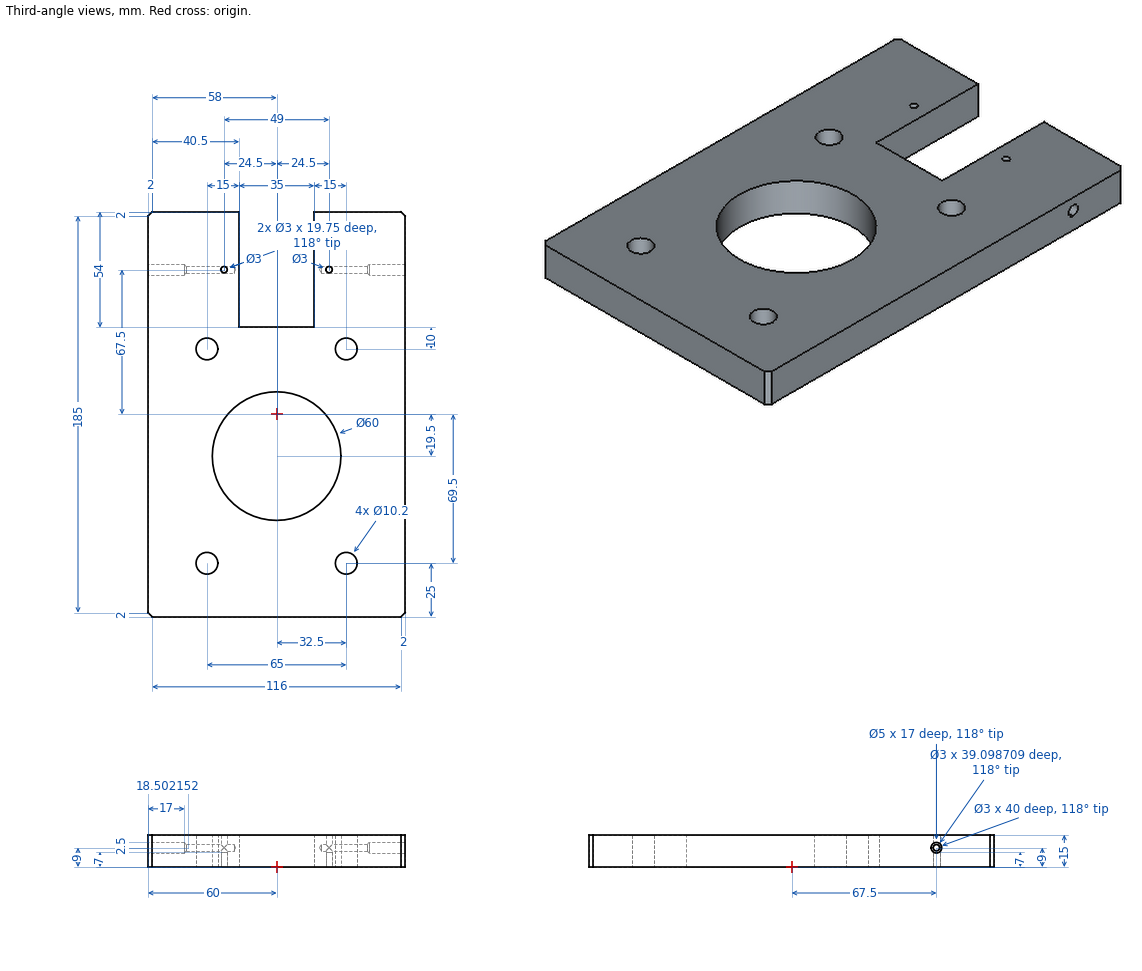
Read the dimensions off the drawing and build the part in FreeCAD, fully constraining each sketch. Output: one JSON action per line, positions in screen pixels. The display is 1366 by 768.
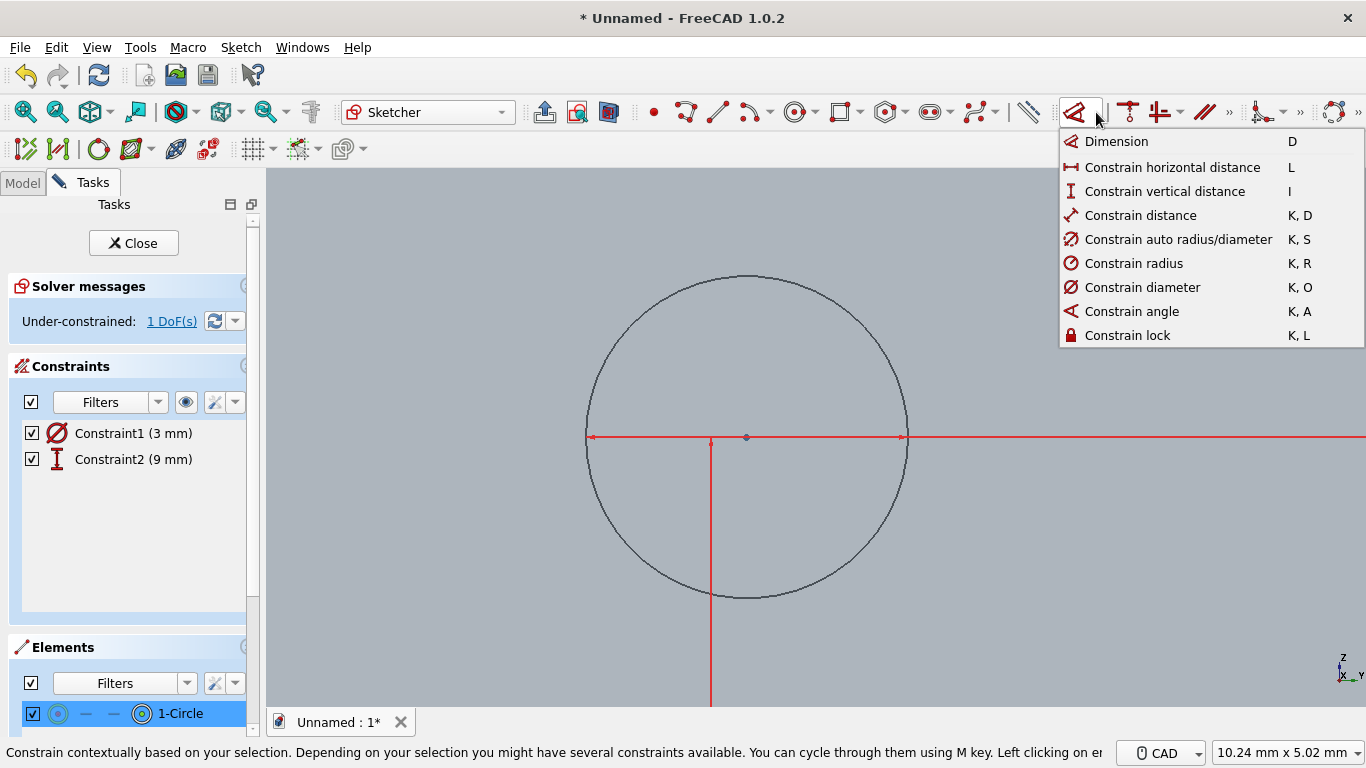
{"action": "left_click", "coordinate": [1212, 167]}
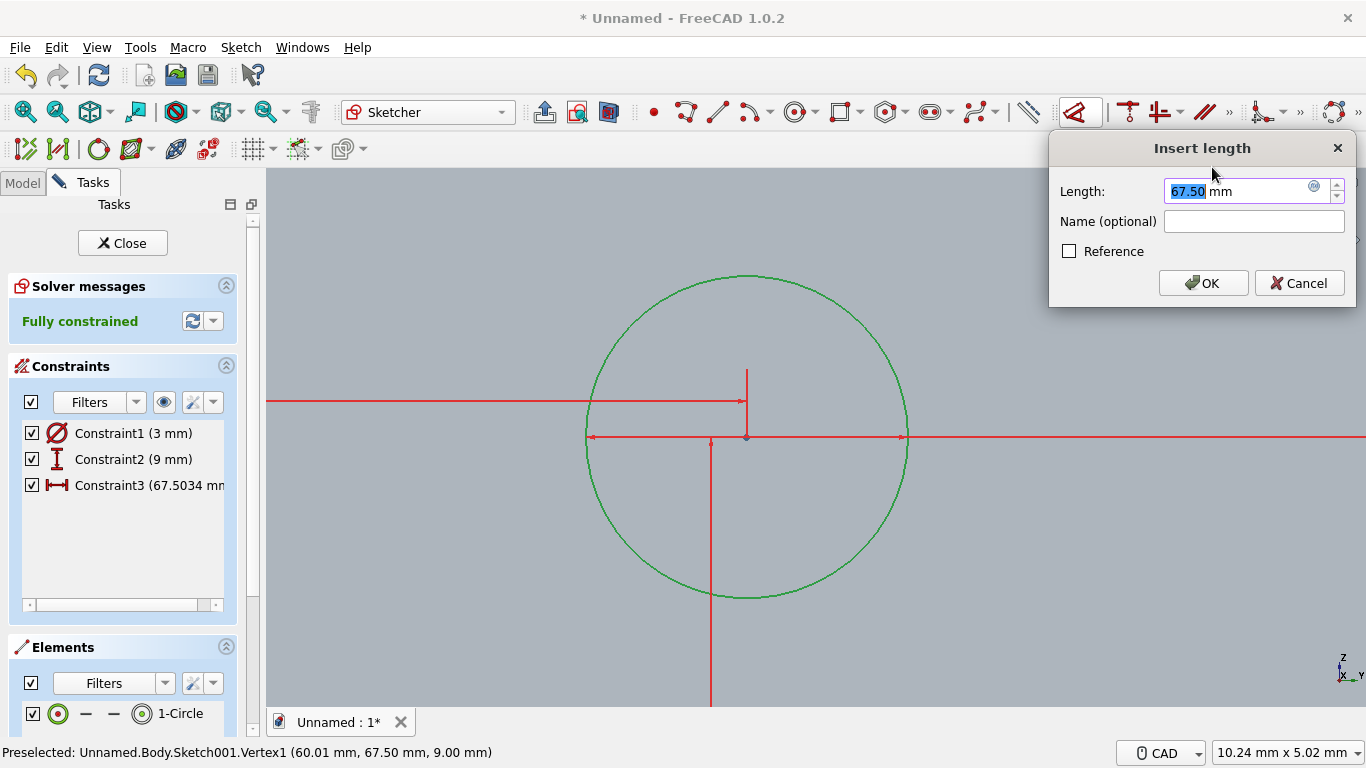
{"action": "type", "text": "67.5"}
{"action": "key", "text": "Return"}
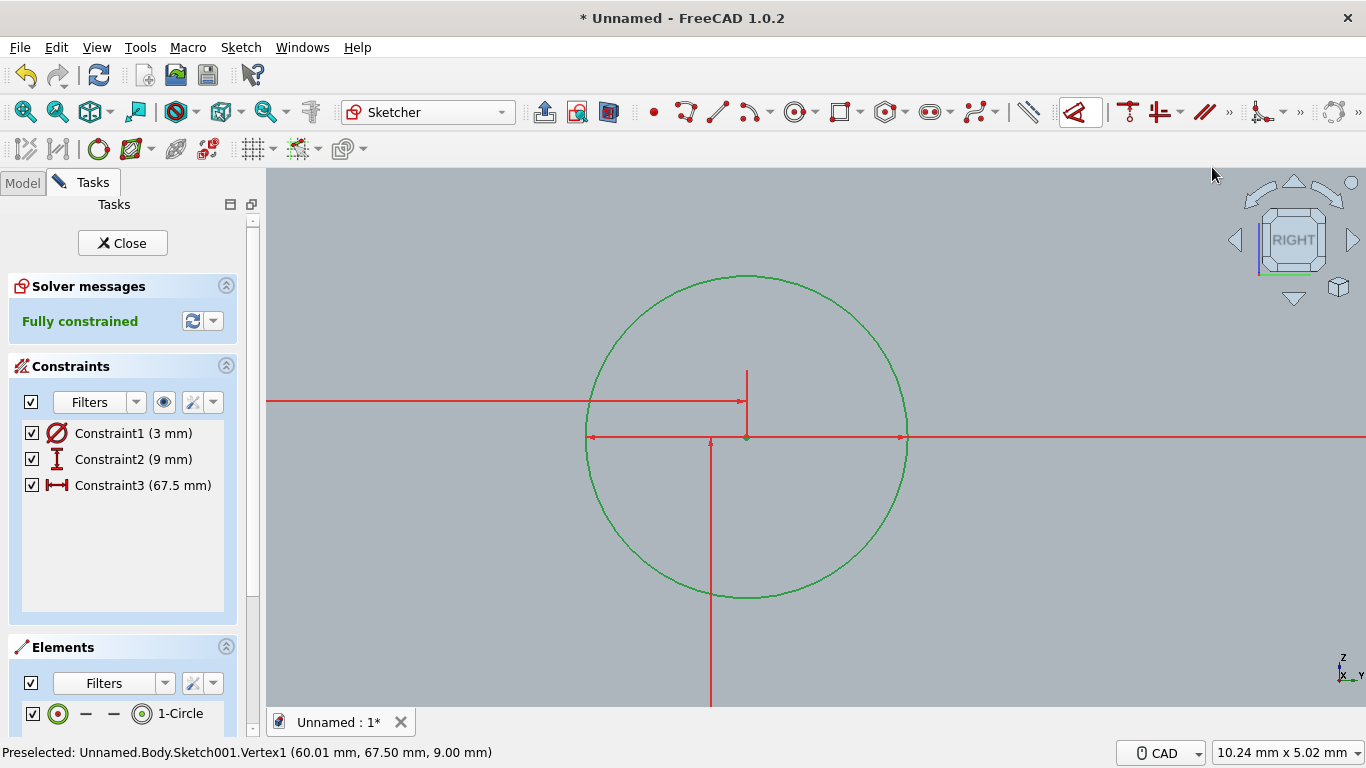
{"action": "left_click", "coordinate": [123, 243]}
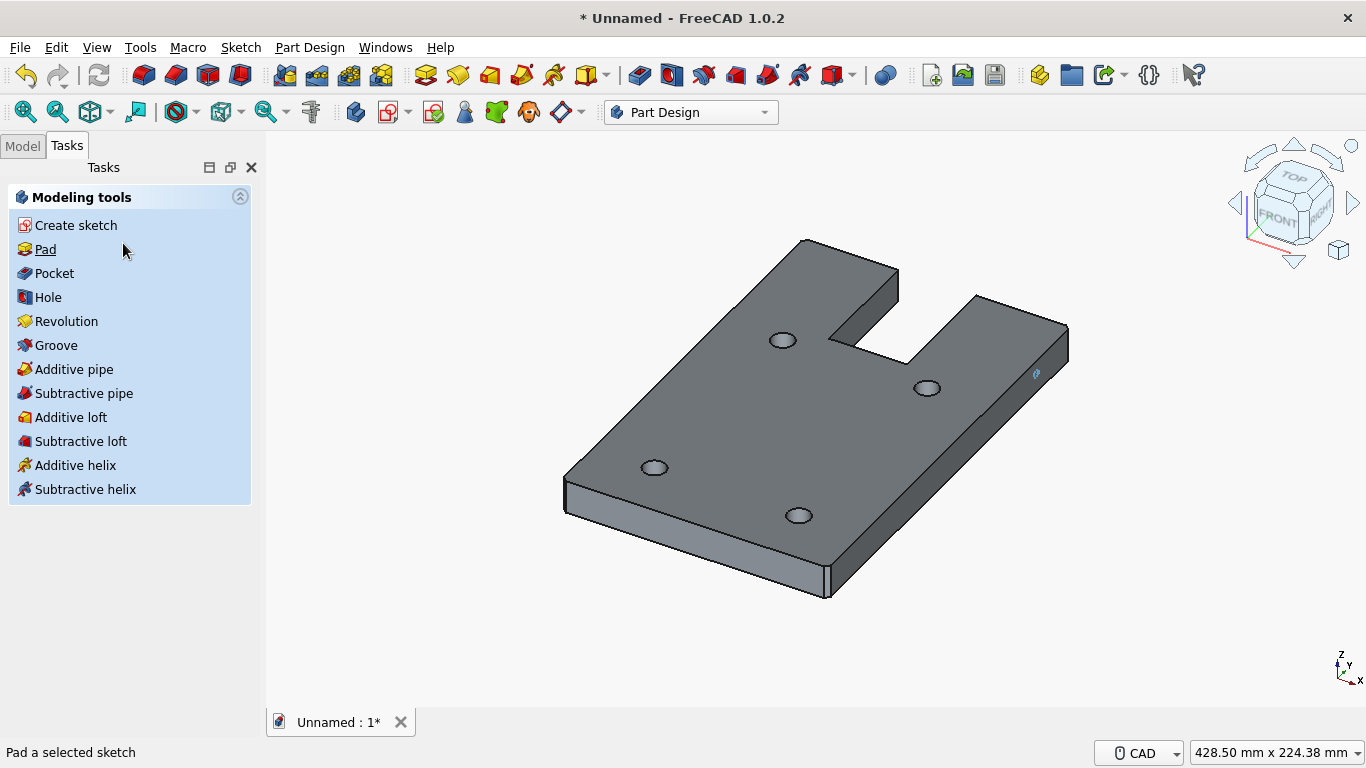
{"action": "left_click", "coordinate": [672, 76]}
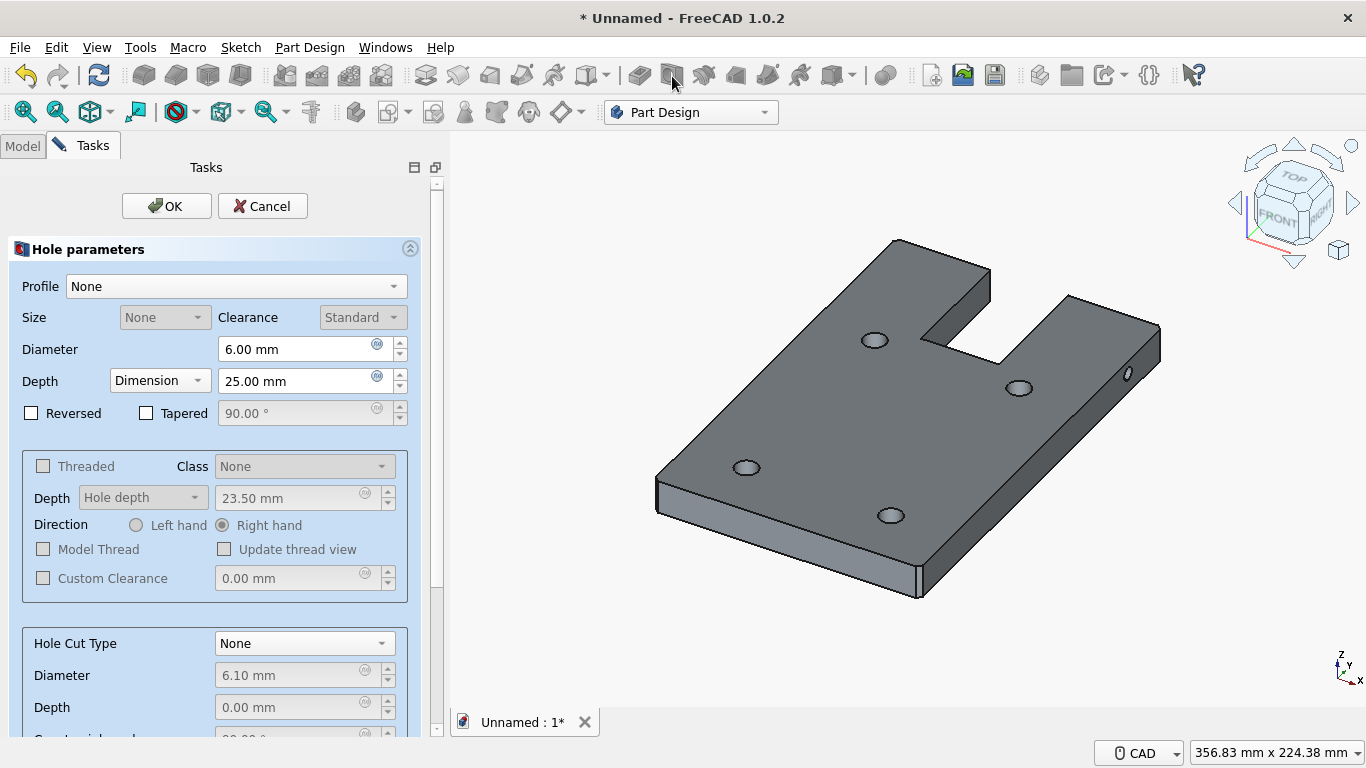
{"action": "triple_click", "coordinate": [305, 349]}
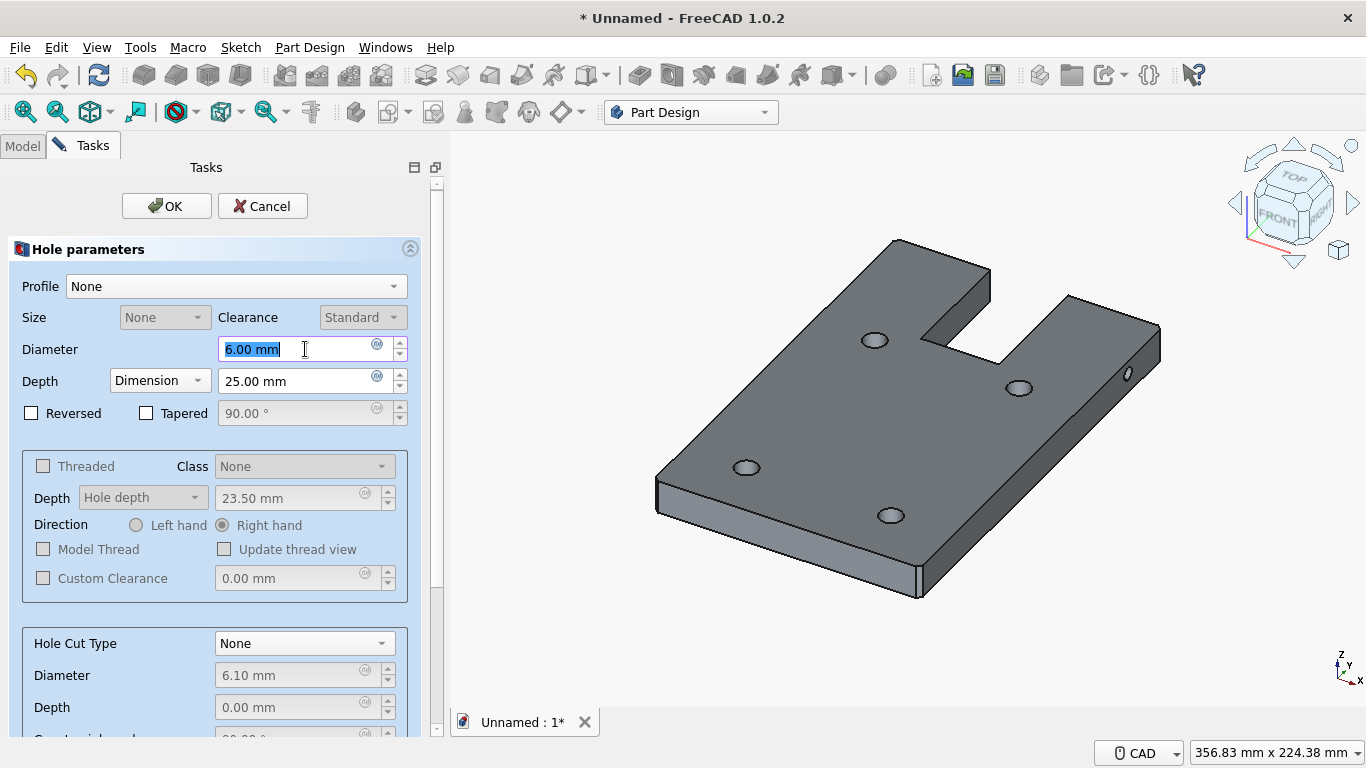
{"action": "type", "text": "3"}
{"action": "key", "text": "Tab"}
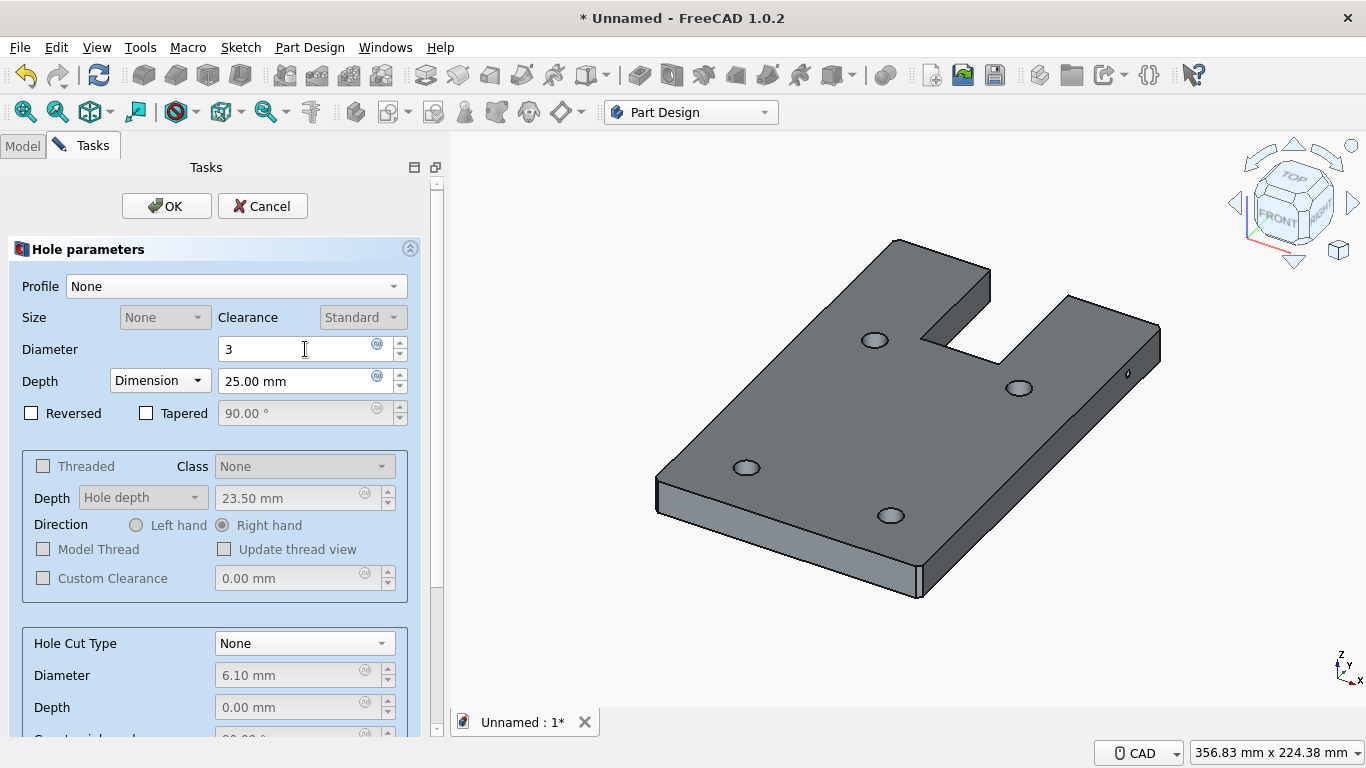
{"action": "triple_click", "coordinate": [305, 381]}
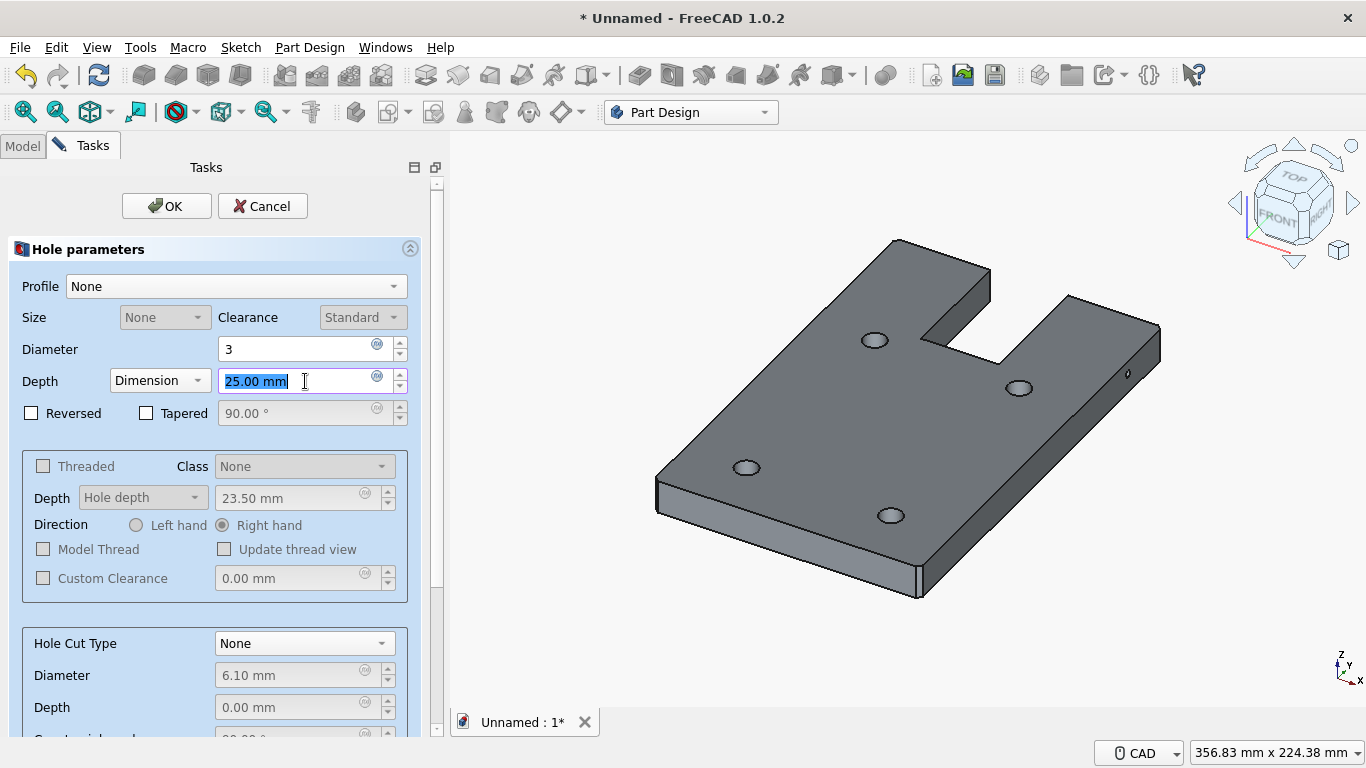
{"action": "type", "text": "39.098709"}
{"action": "key", "text": "Tab"}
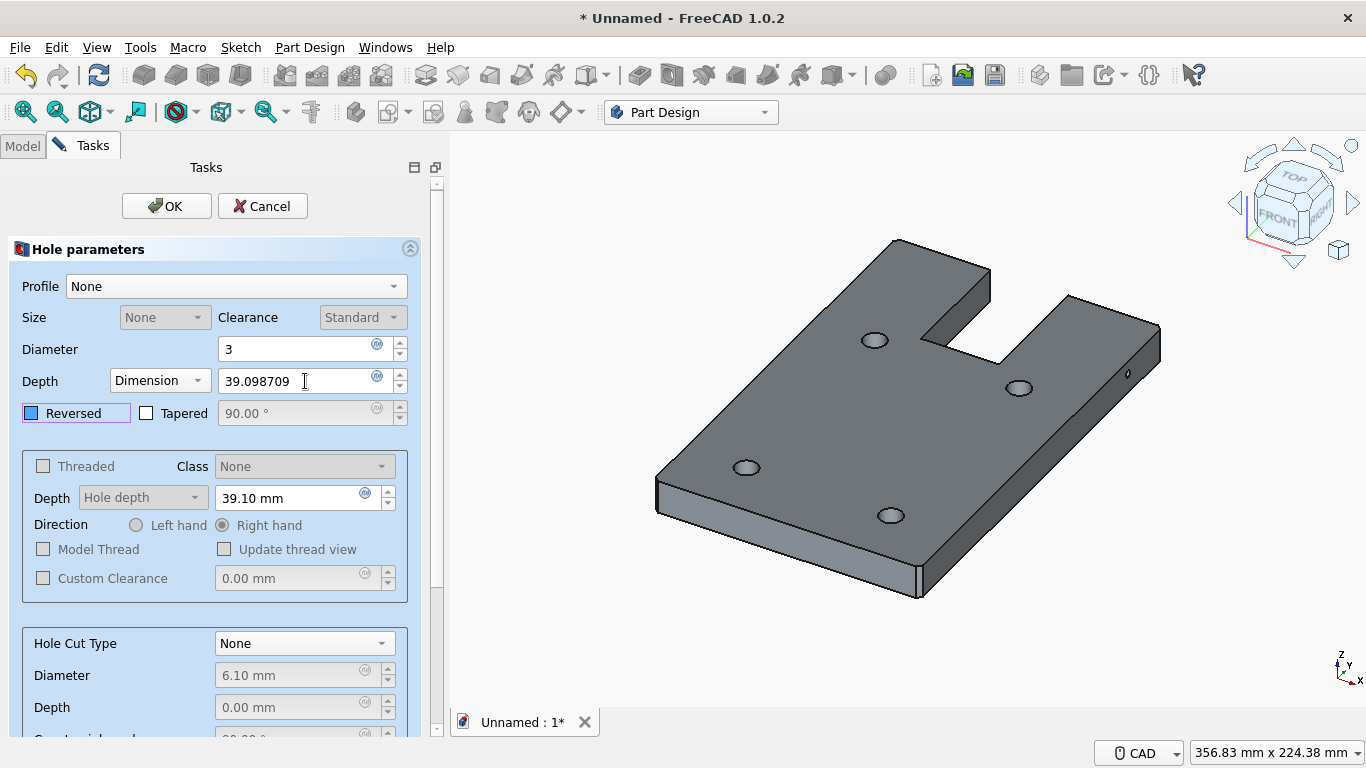
{"action": "left_click", "coordinate": [167, 206]}